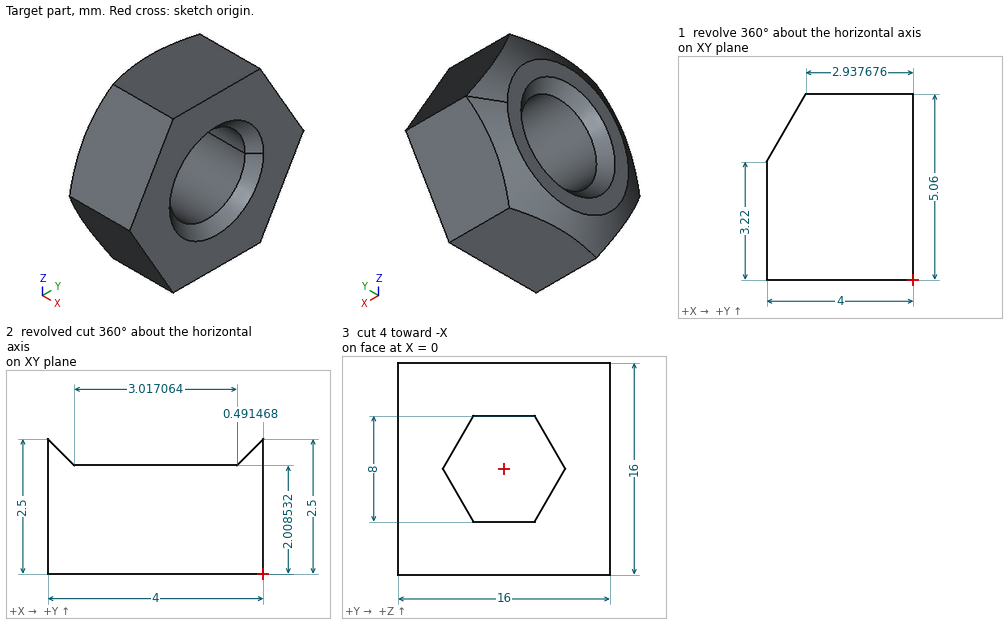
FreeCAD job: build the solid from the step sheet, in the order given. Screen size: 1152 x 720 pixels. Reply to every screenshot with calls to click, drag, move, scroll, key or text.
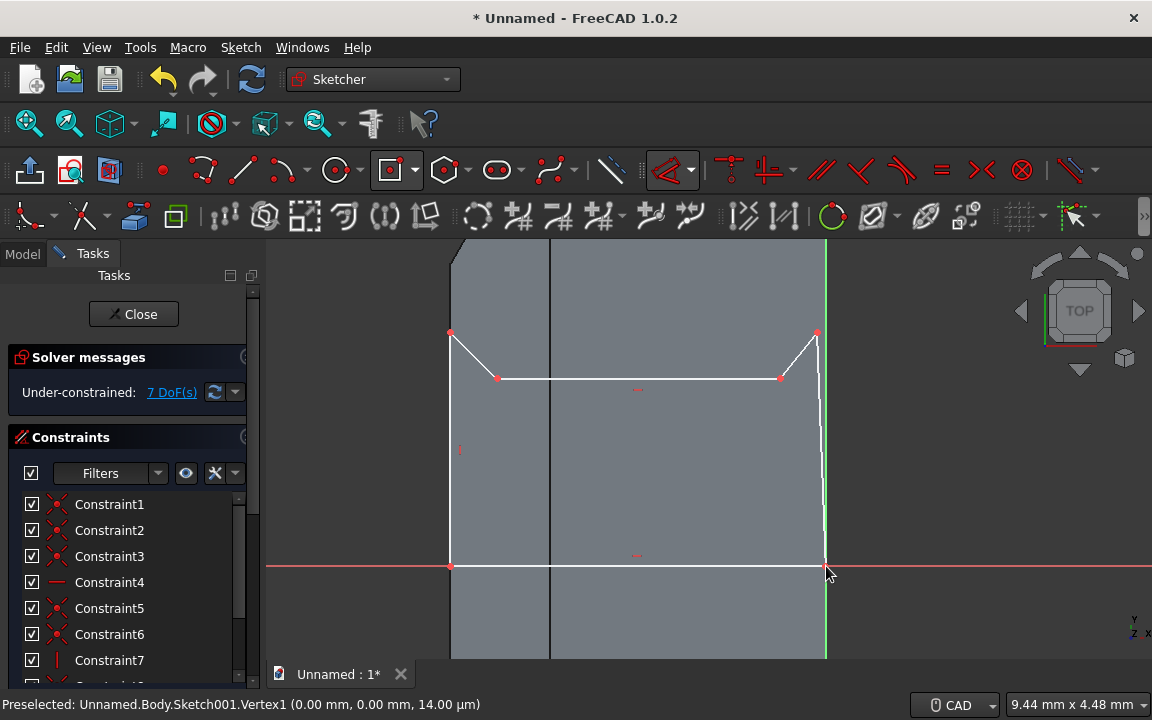
click(823, 496)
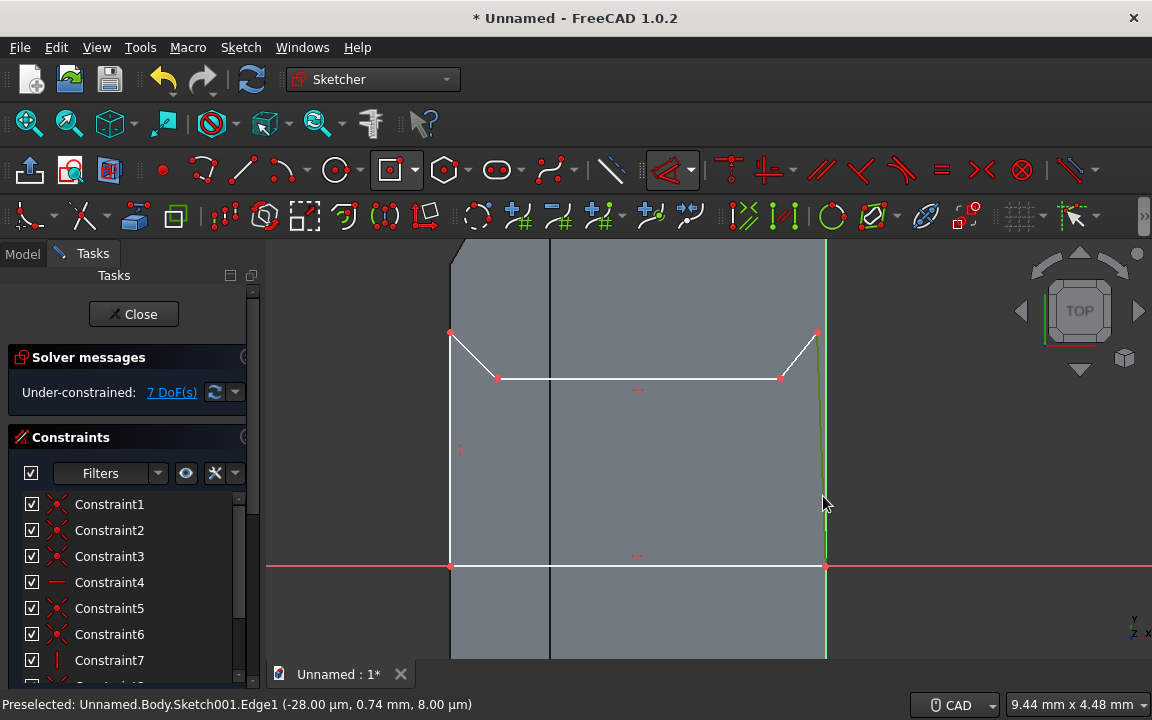
key(v)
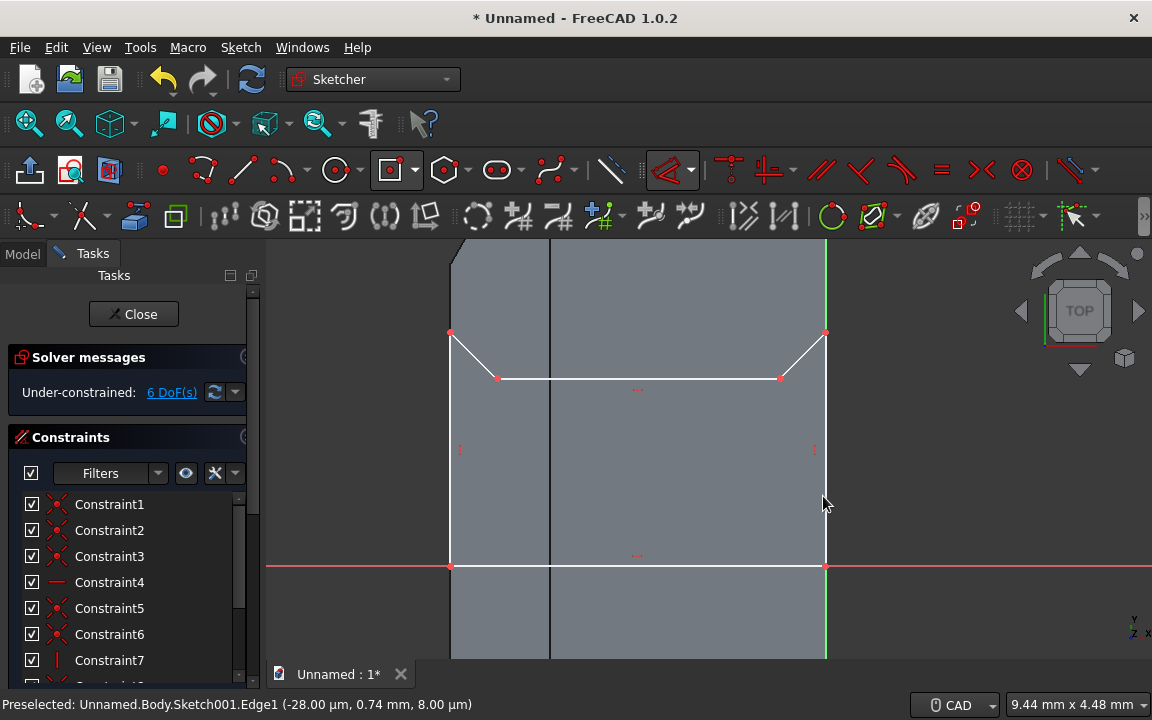
click(563, 566)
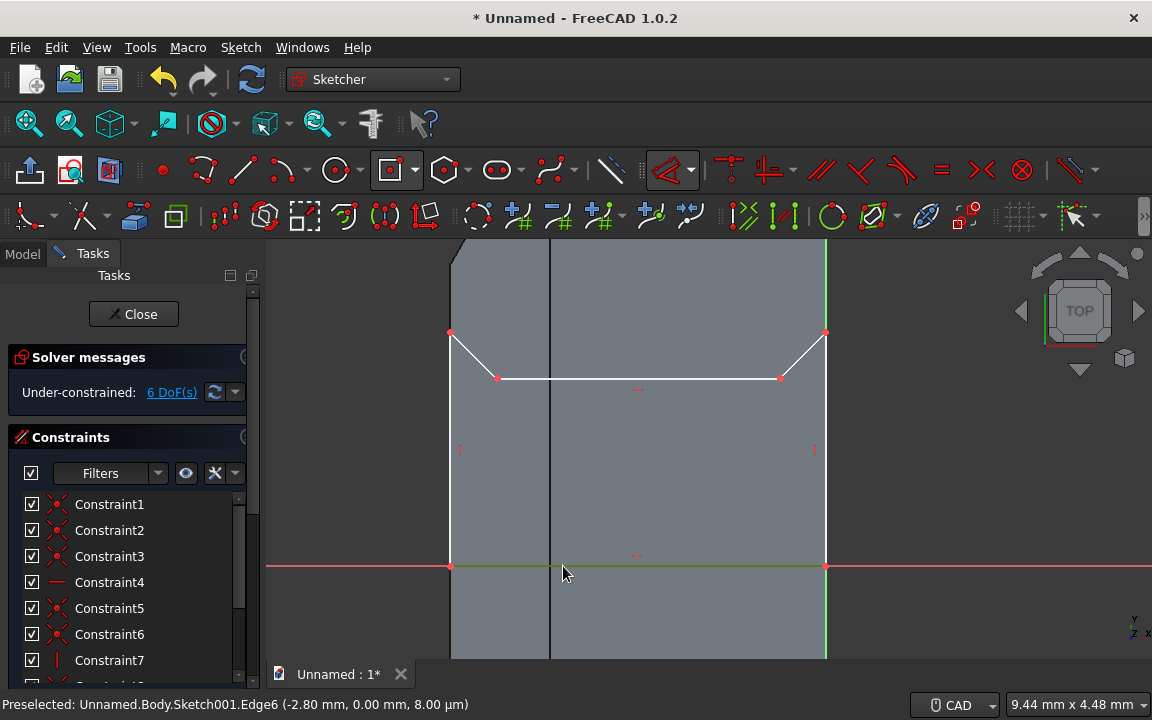
key(l)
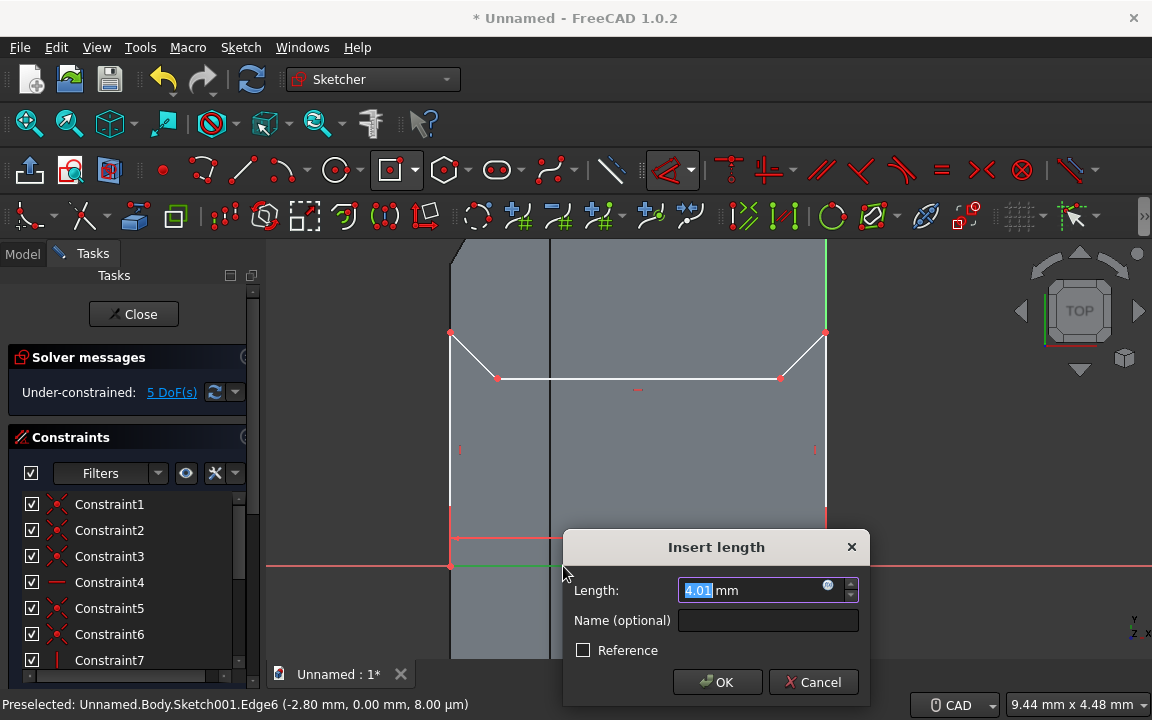
text(4)
key(Return)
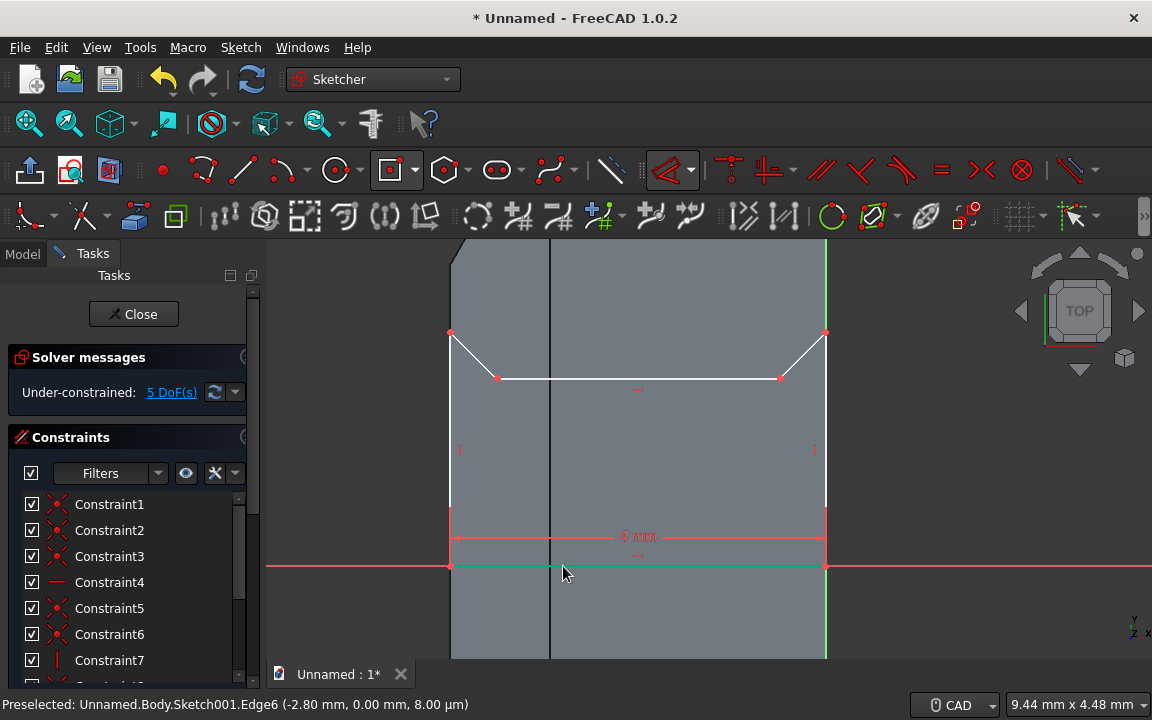
click(826, 496)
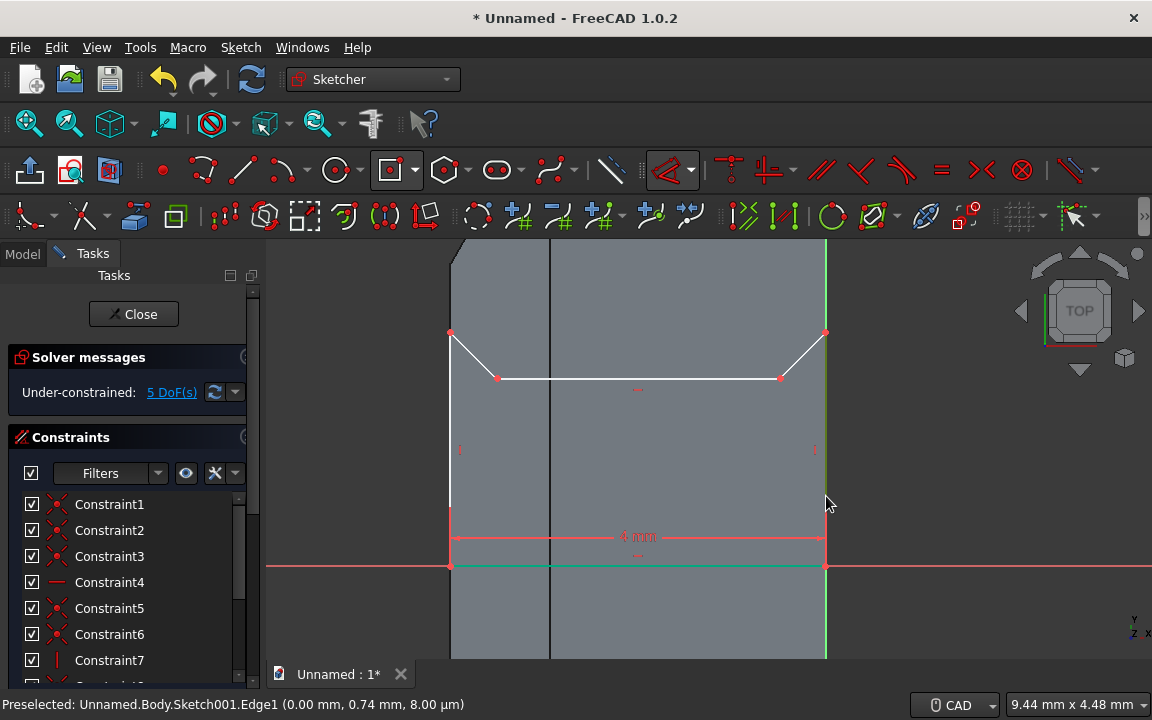
key(i)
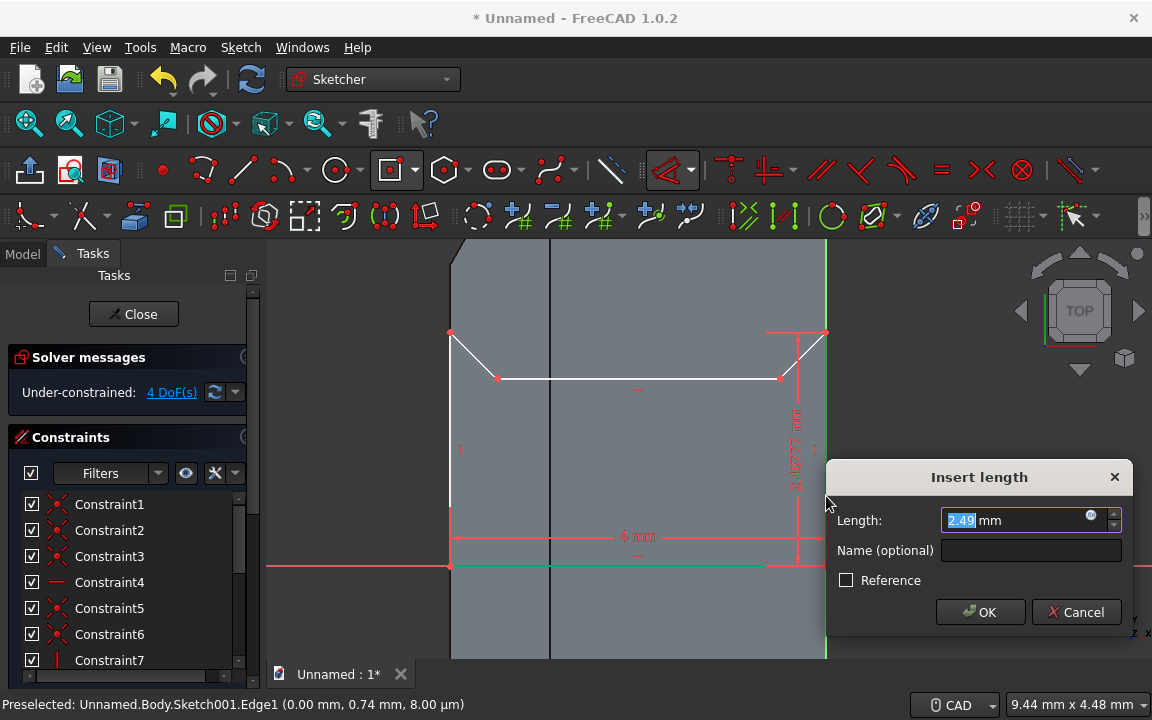
text(2.5)
key(Return)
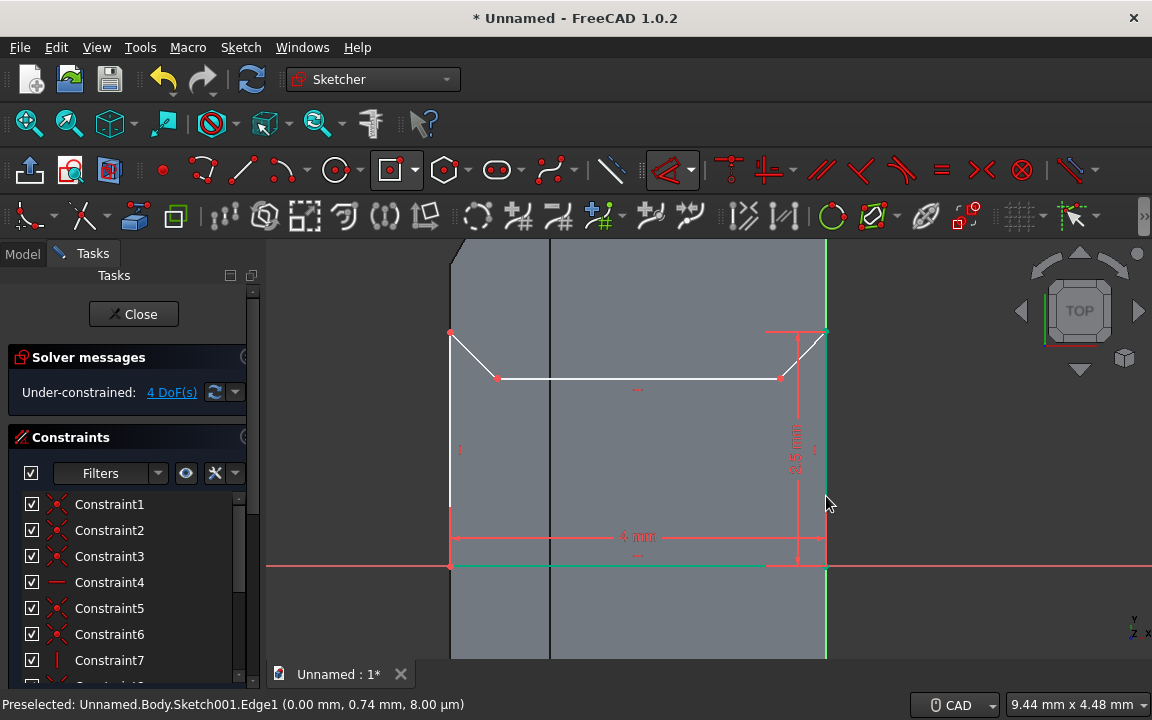
click(450, 403)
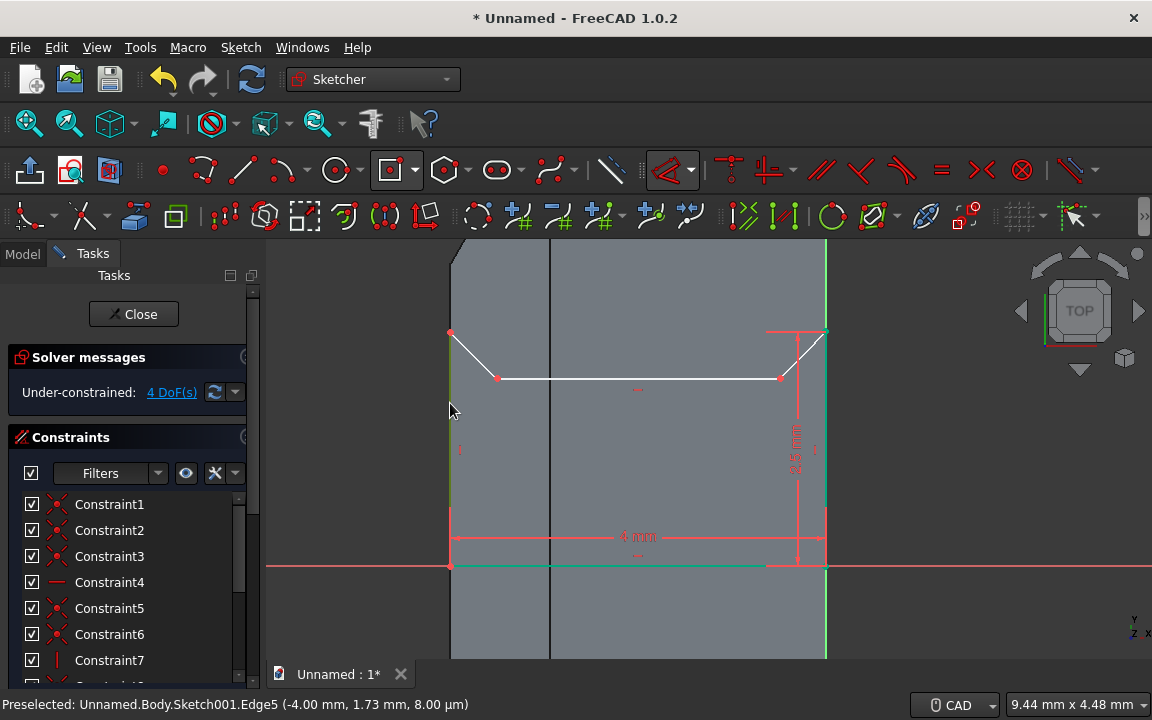
key(i)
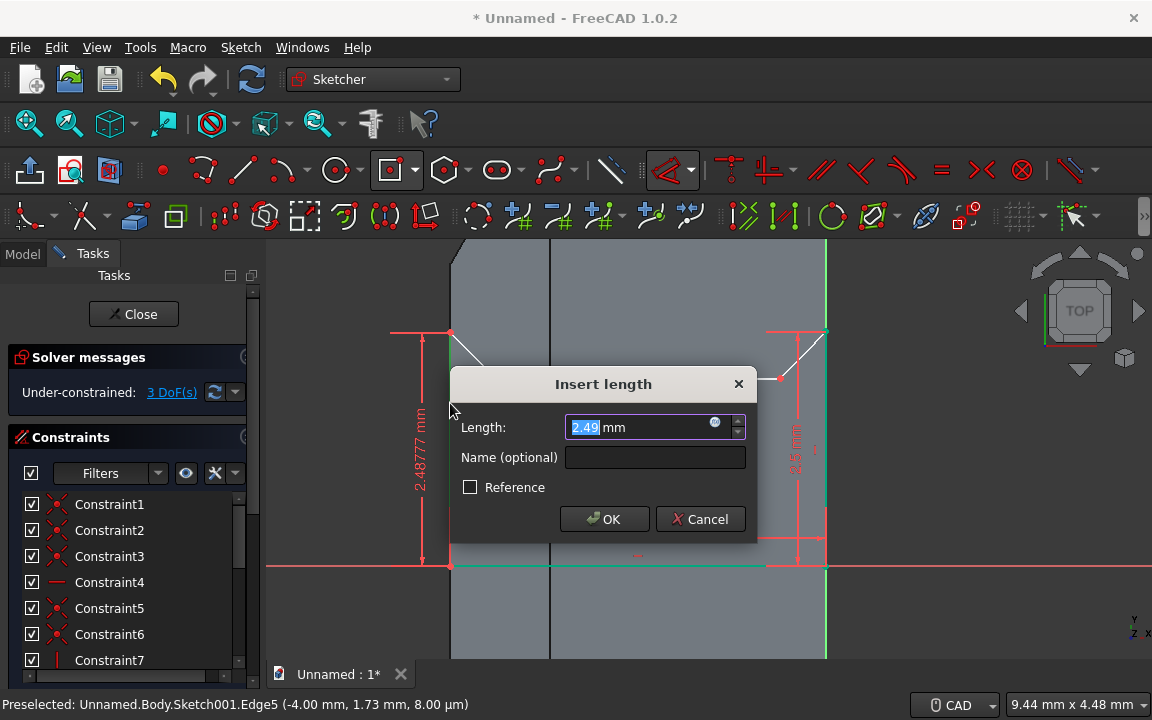
text(2.5)
key(Return)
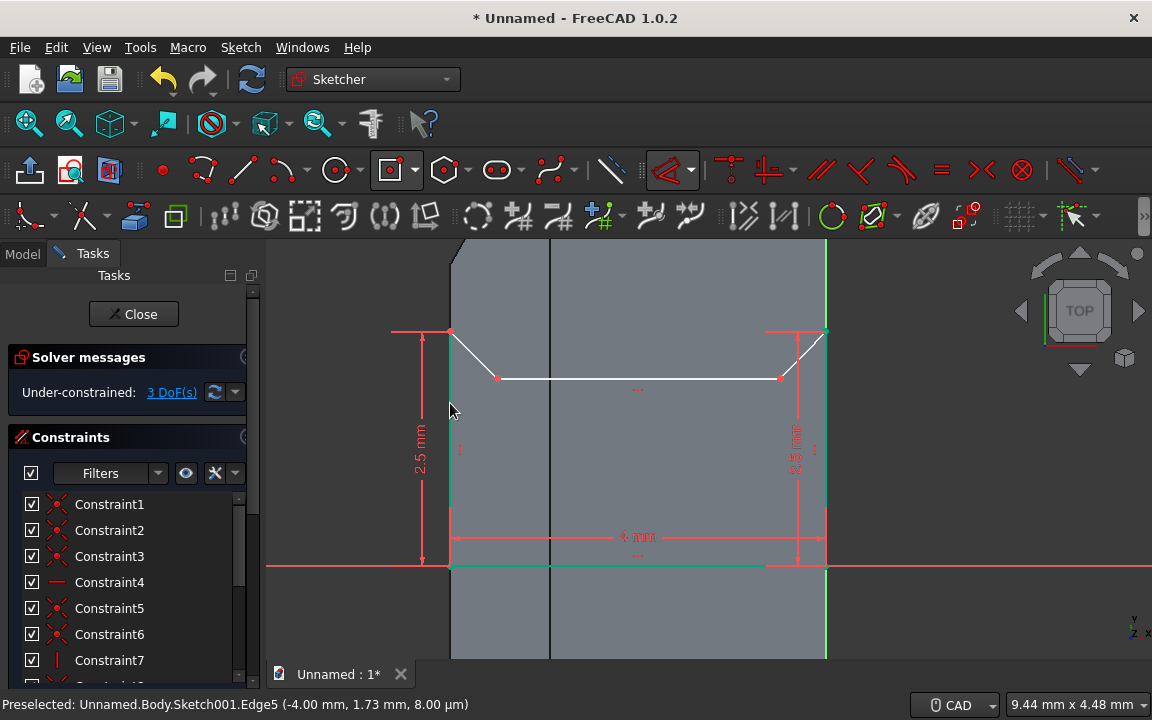
click(695, 379)